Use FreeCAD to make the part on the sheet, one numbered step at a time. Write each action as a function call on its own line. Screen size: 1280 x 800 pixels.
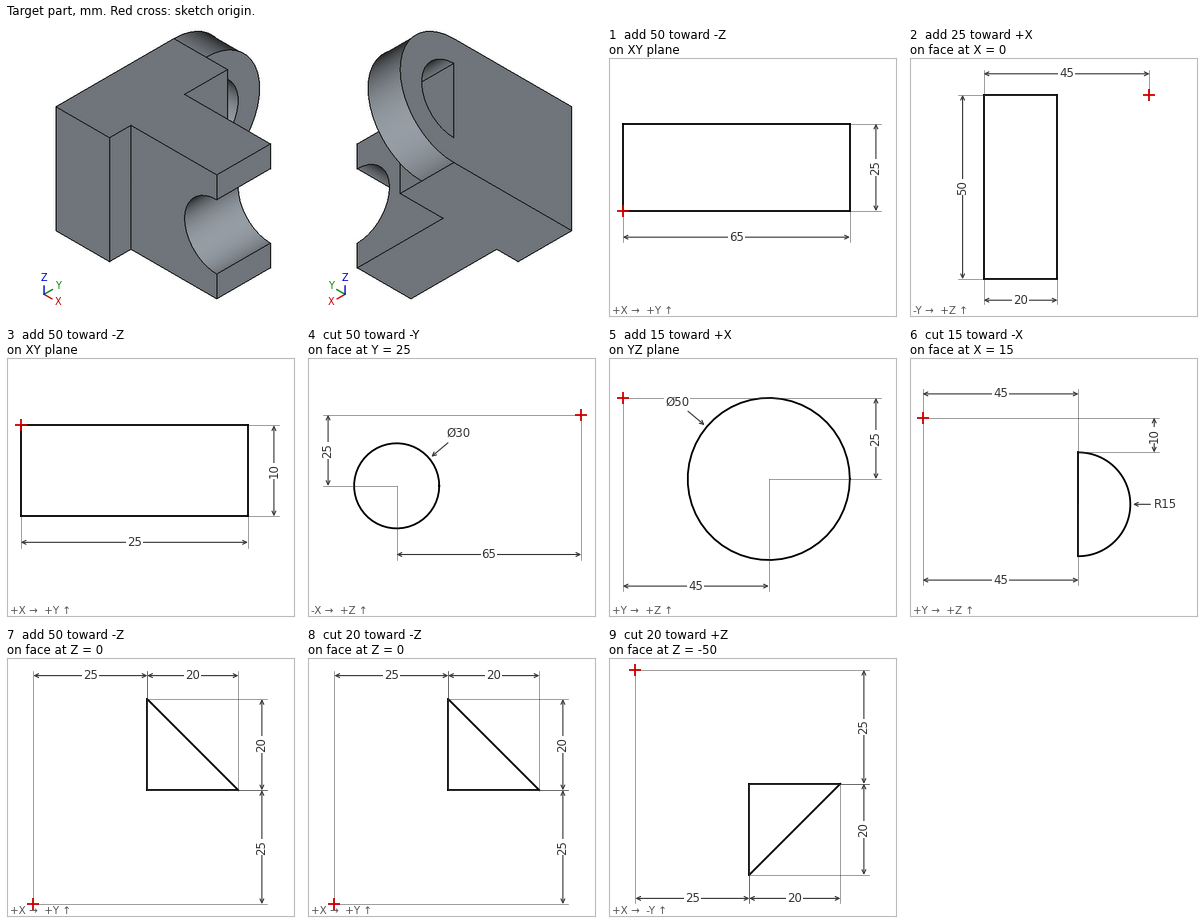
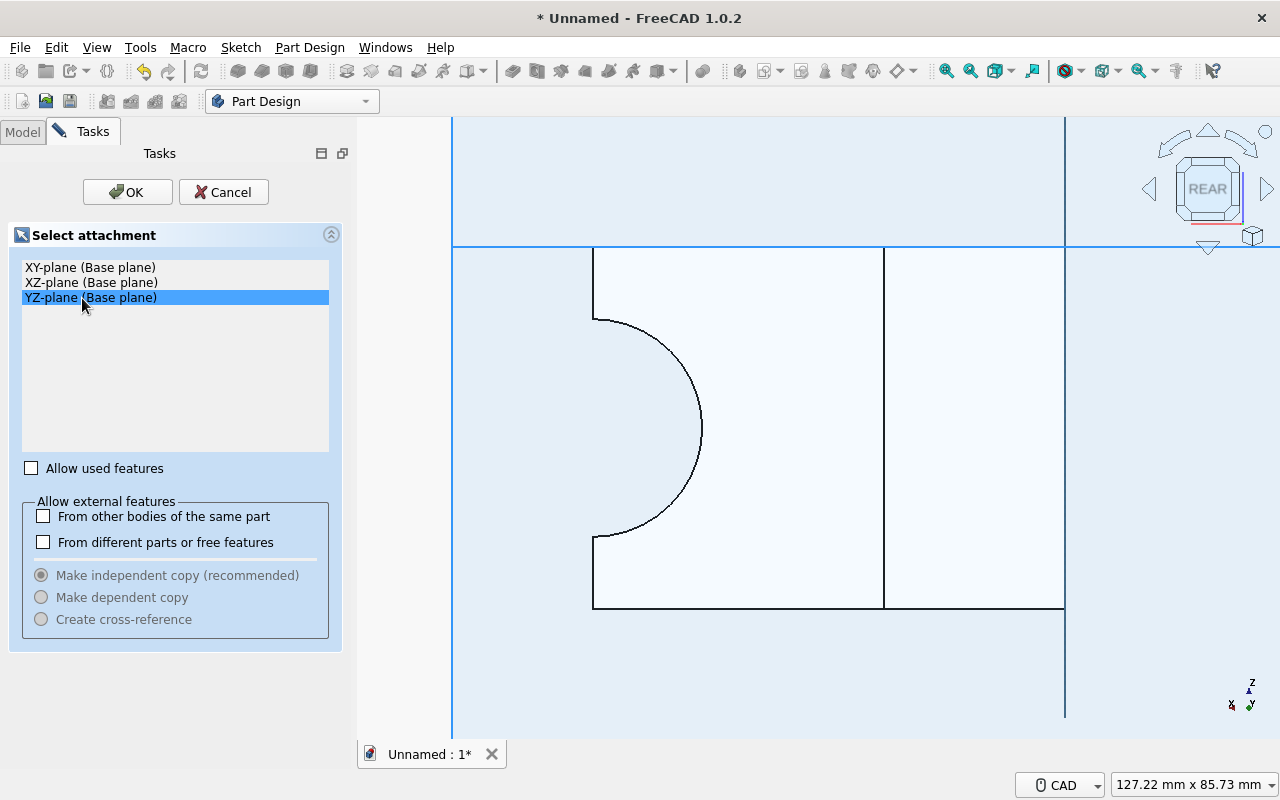
click(128, 192)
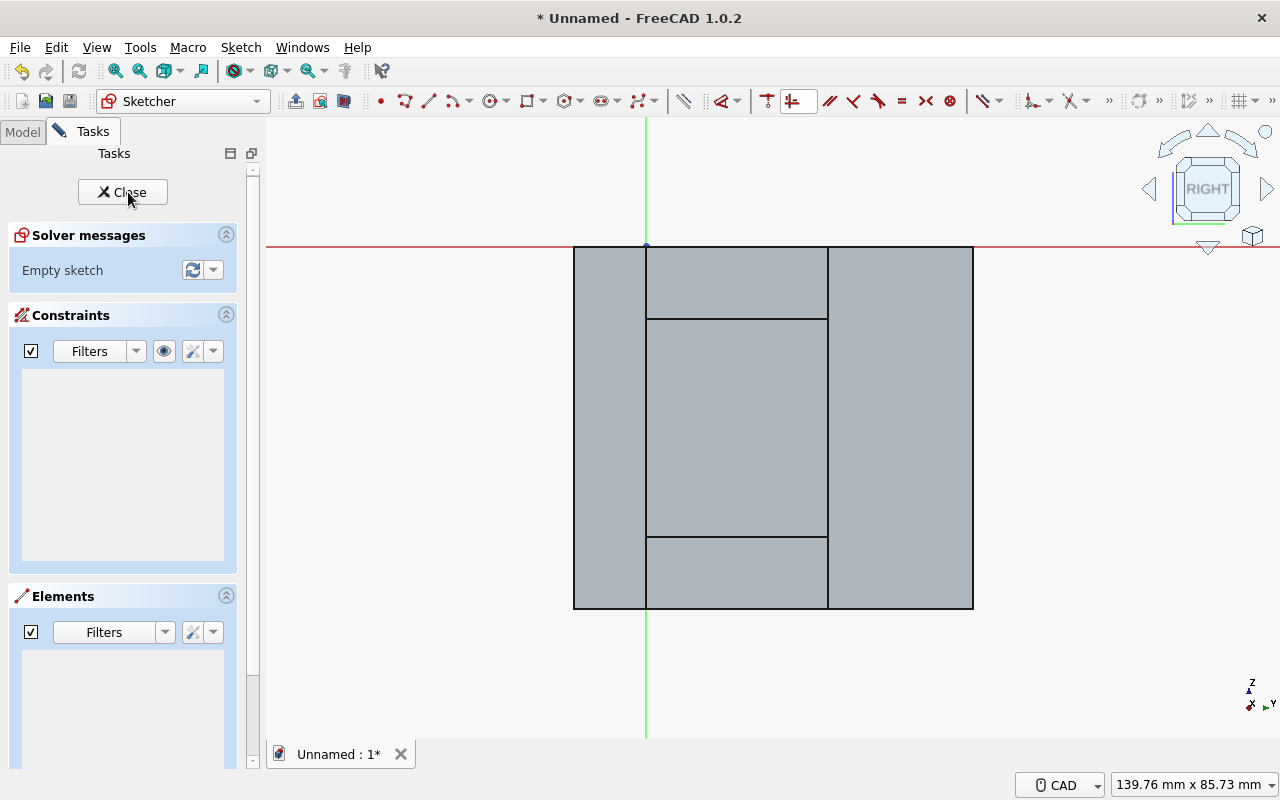
click(344, 102)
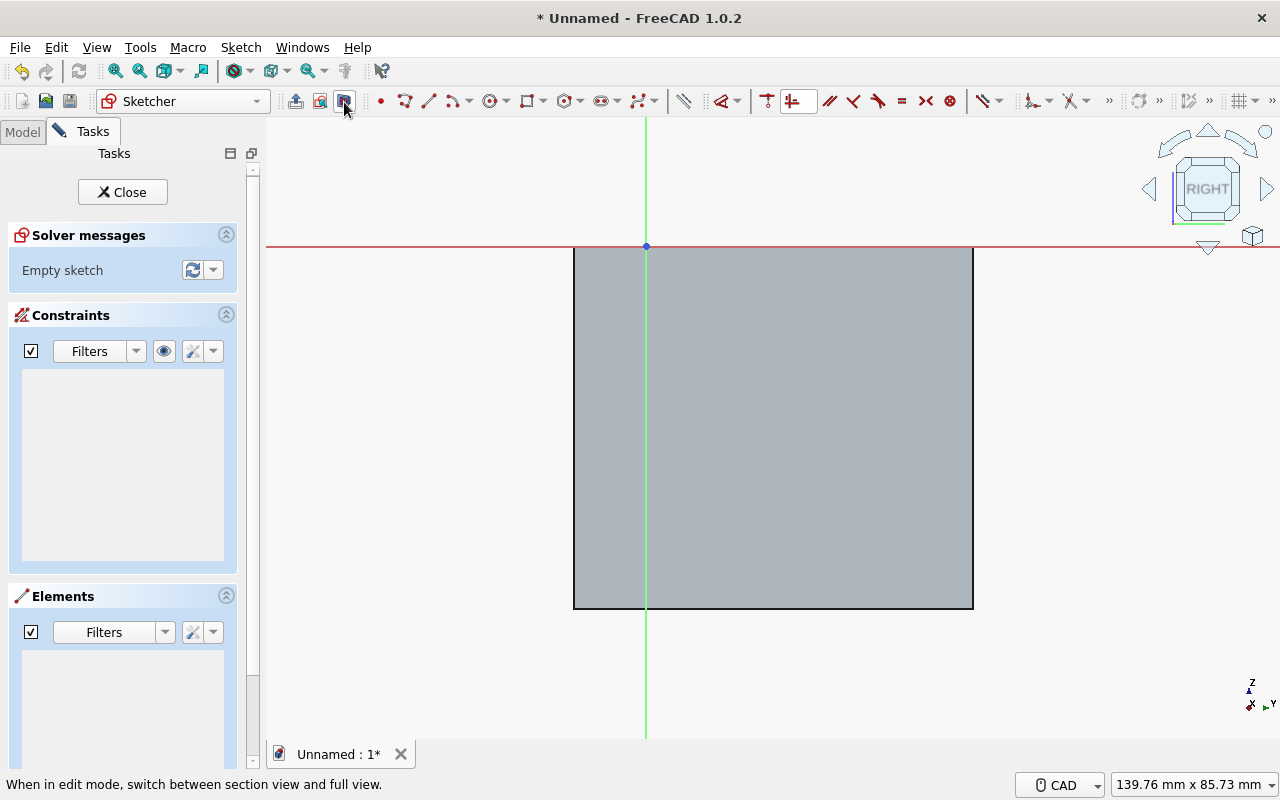
scroll(294, 428, down, 1)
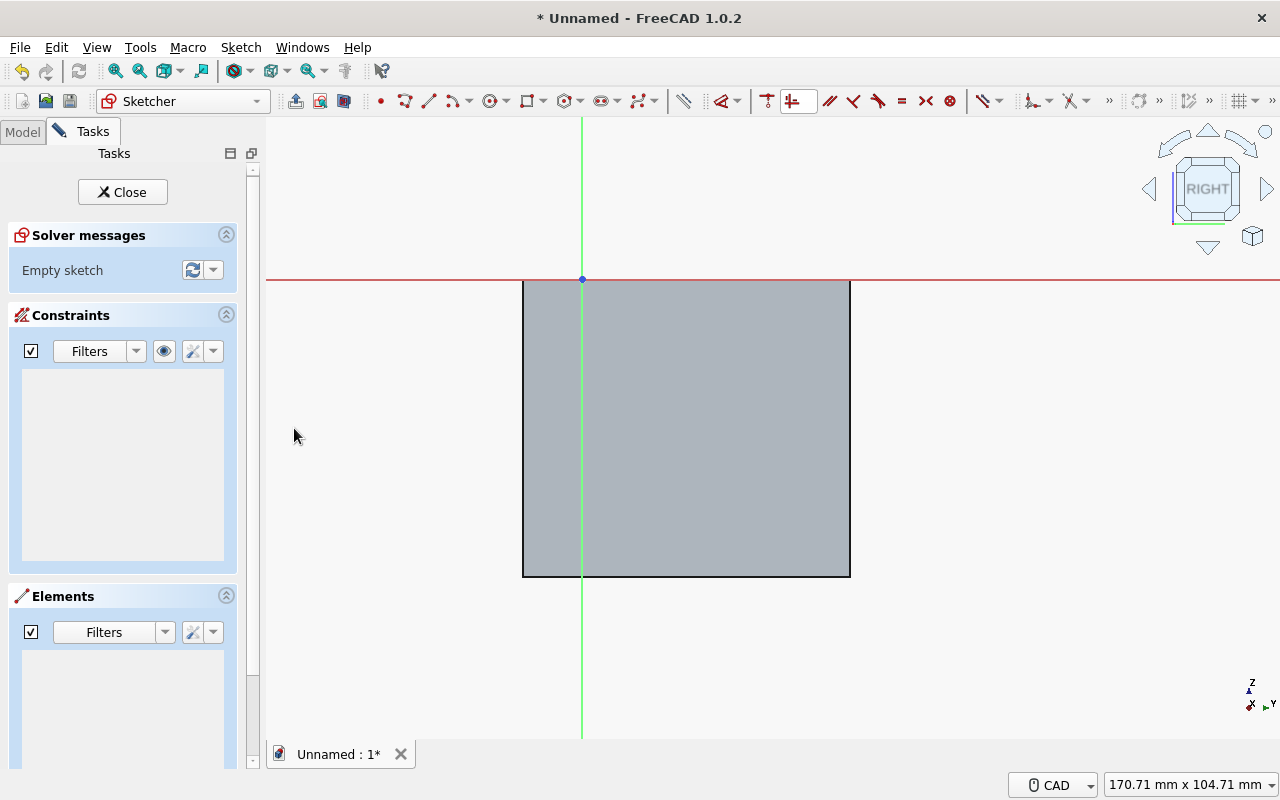
click(490, 102)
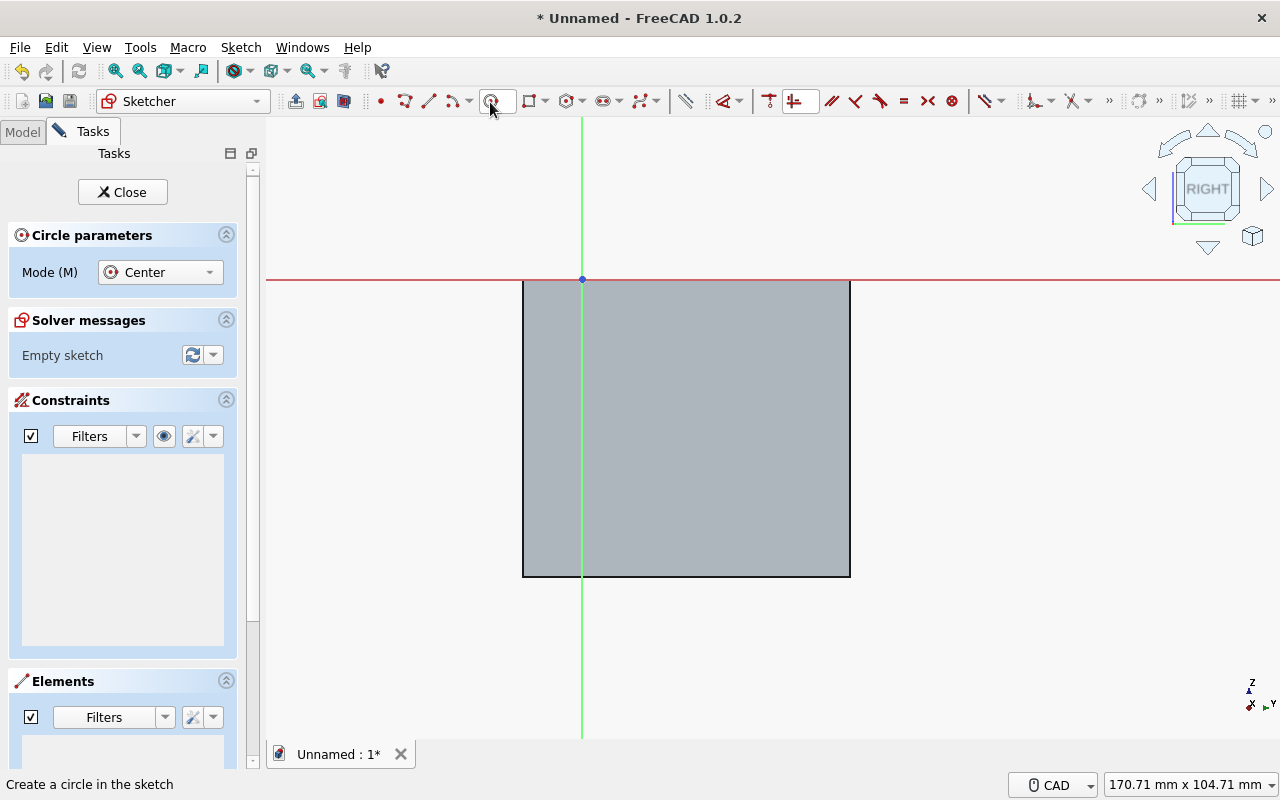
click(850, 428)
move(955, 323)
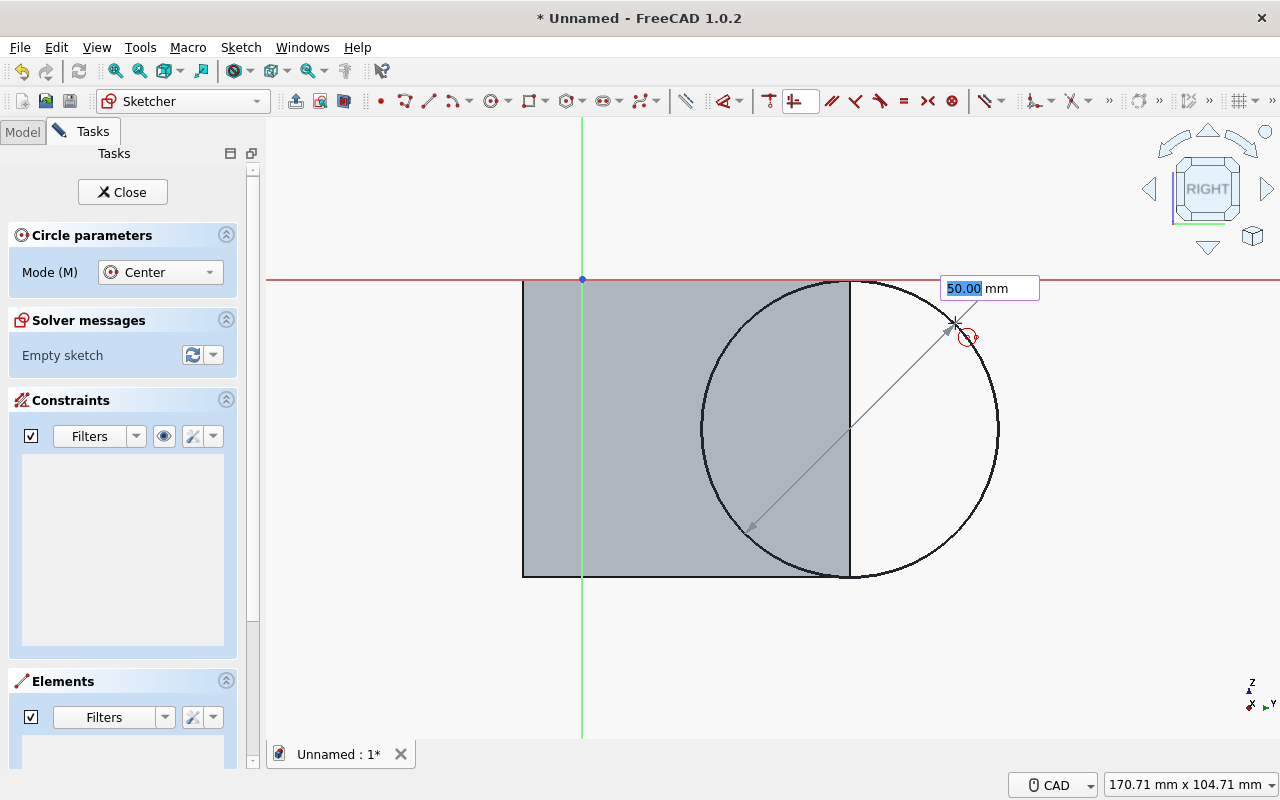
text(50)
key(Return)
key(Escape)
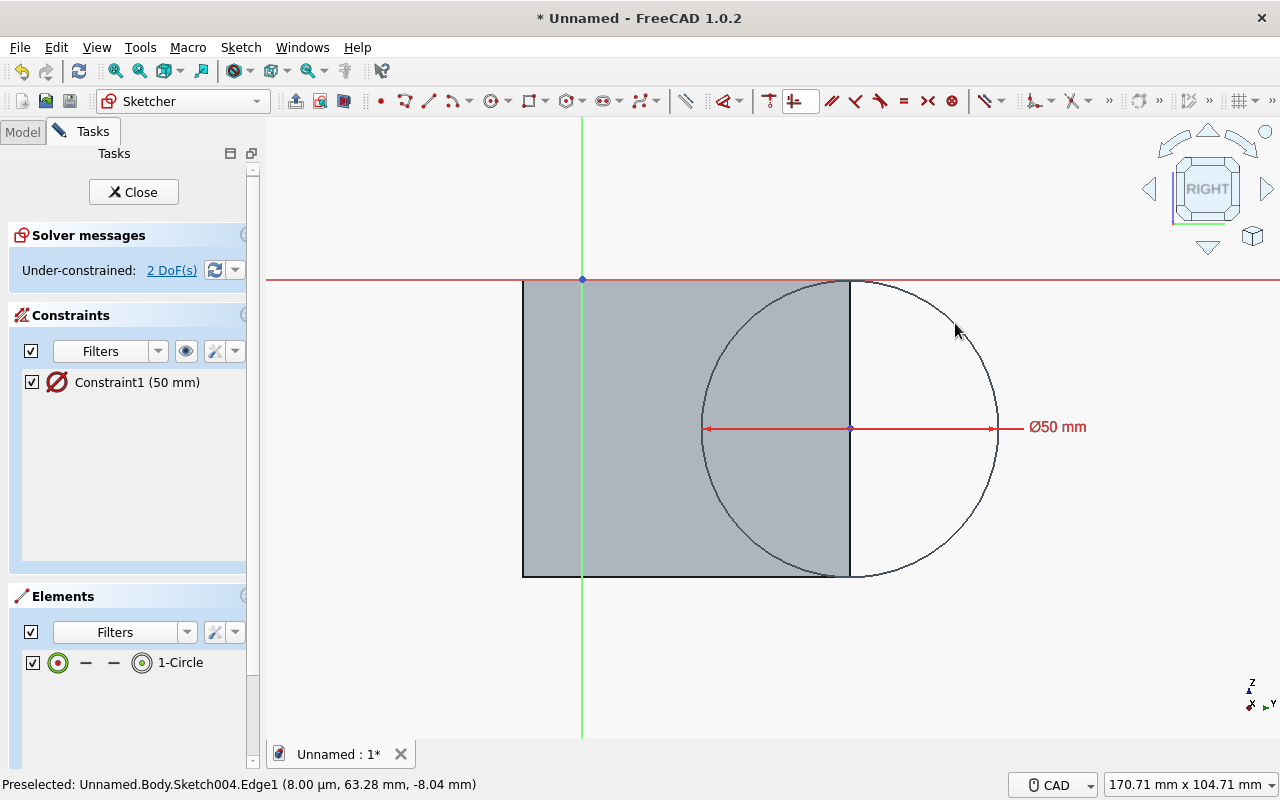
click(850, 429)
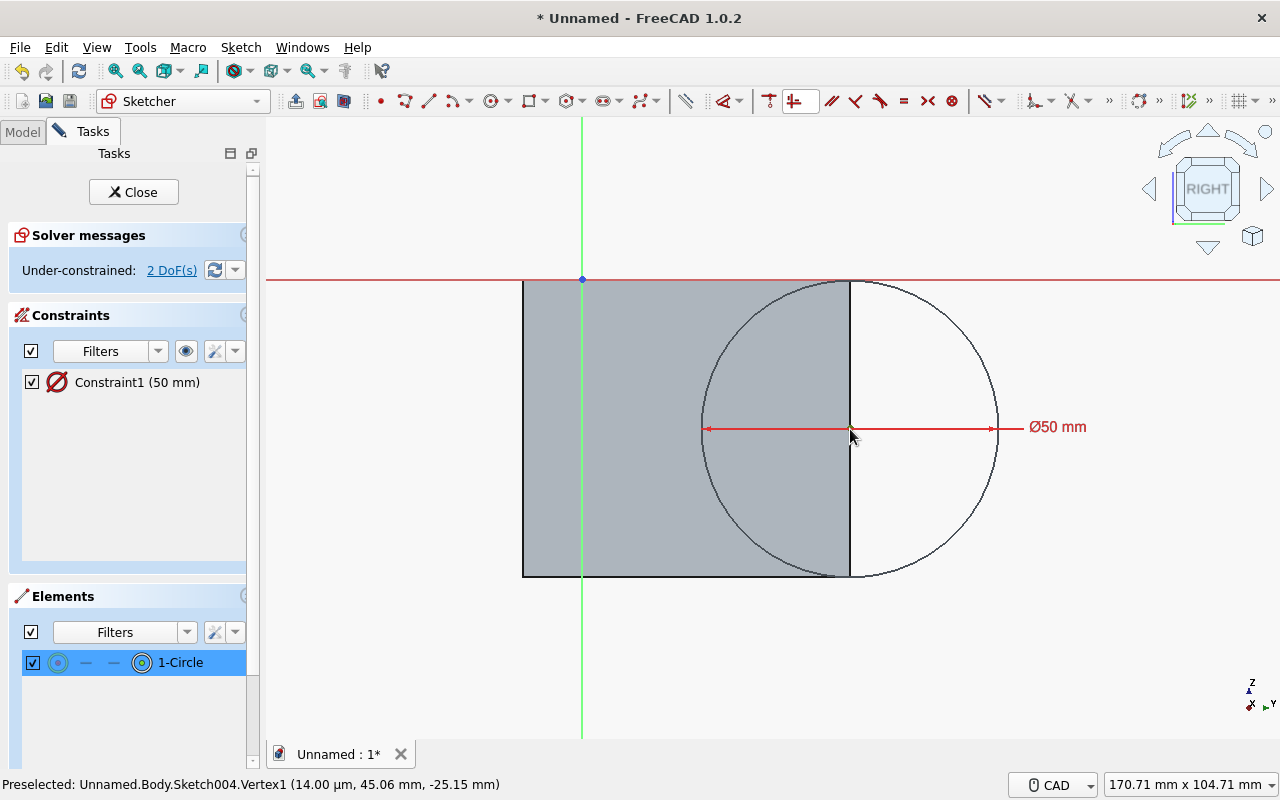
click(742, 102)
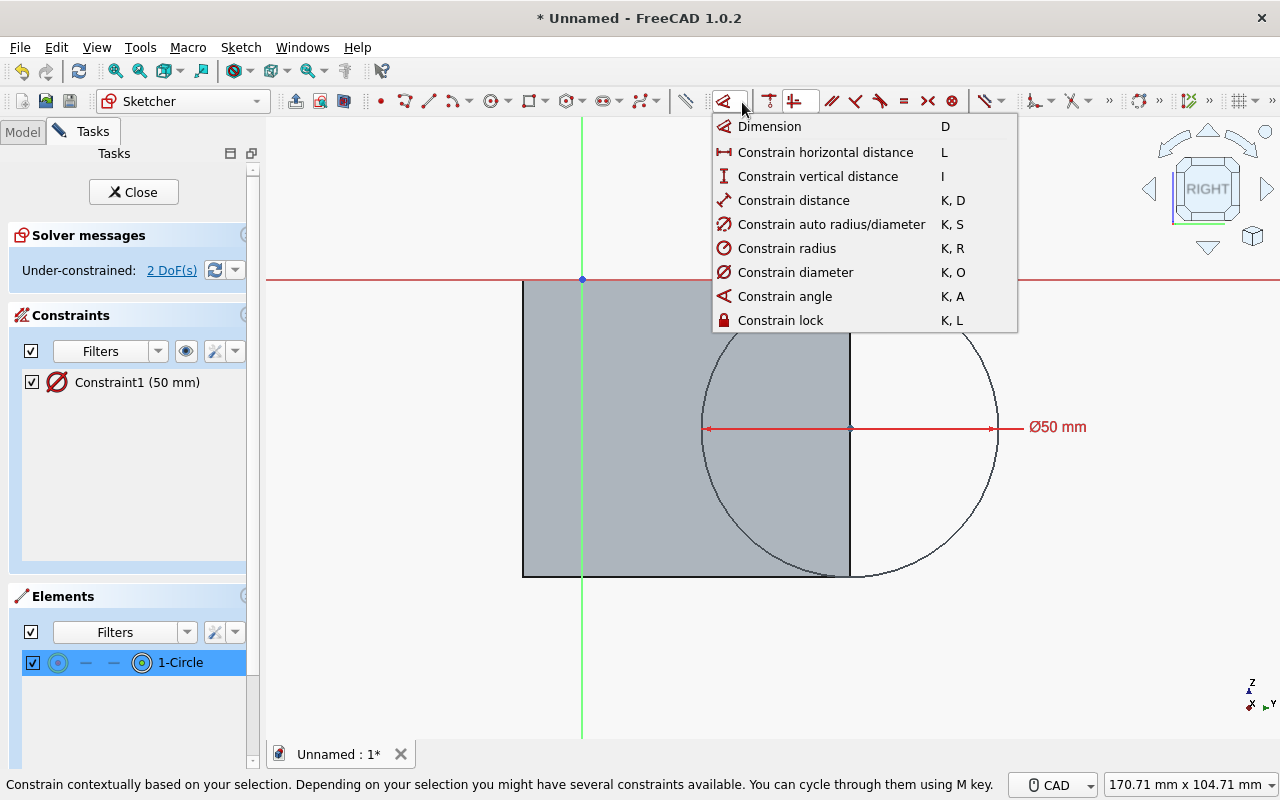
click(865, 152)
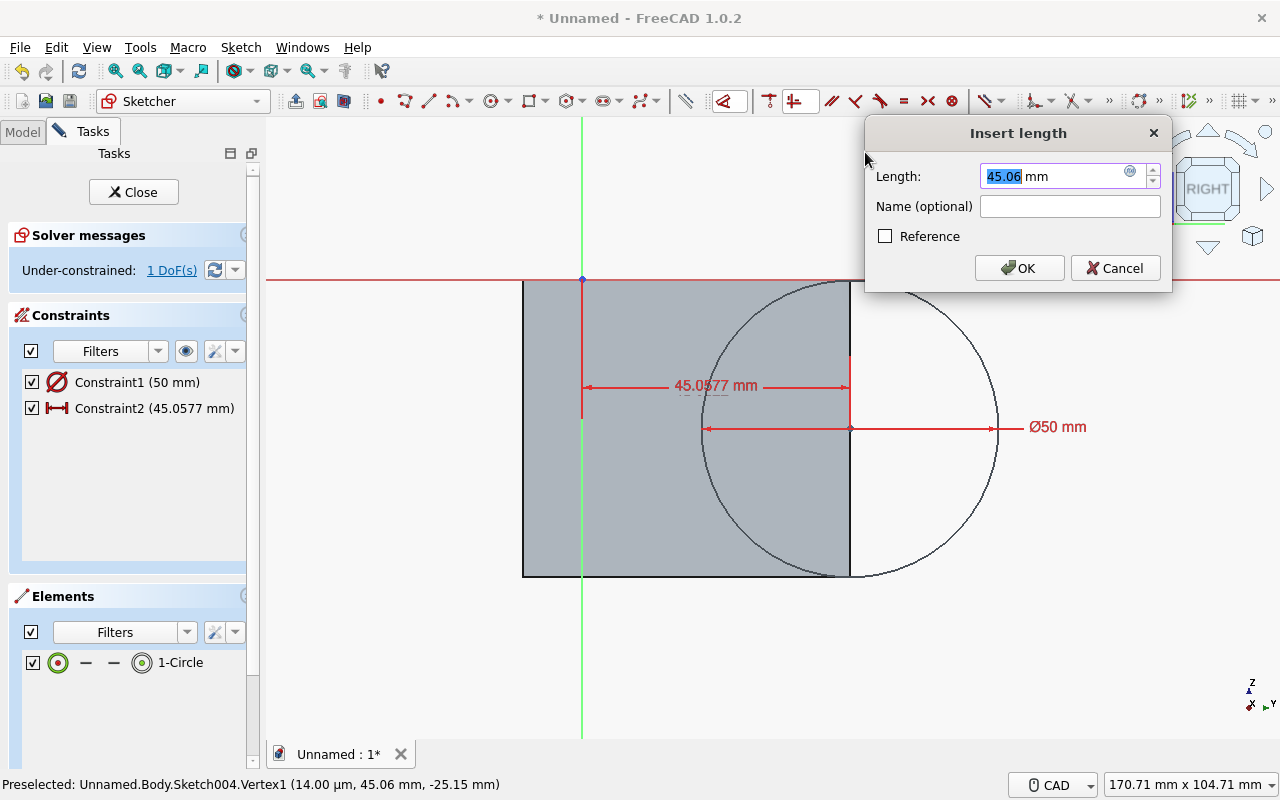
text(45)
key(Return)